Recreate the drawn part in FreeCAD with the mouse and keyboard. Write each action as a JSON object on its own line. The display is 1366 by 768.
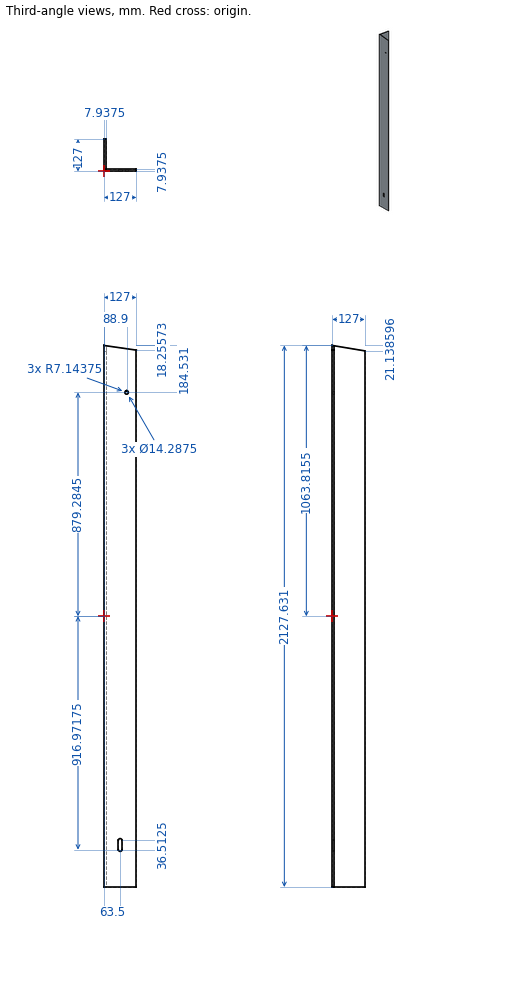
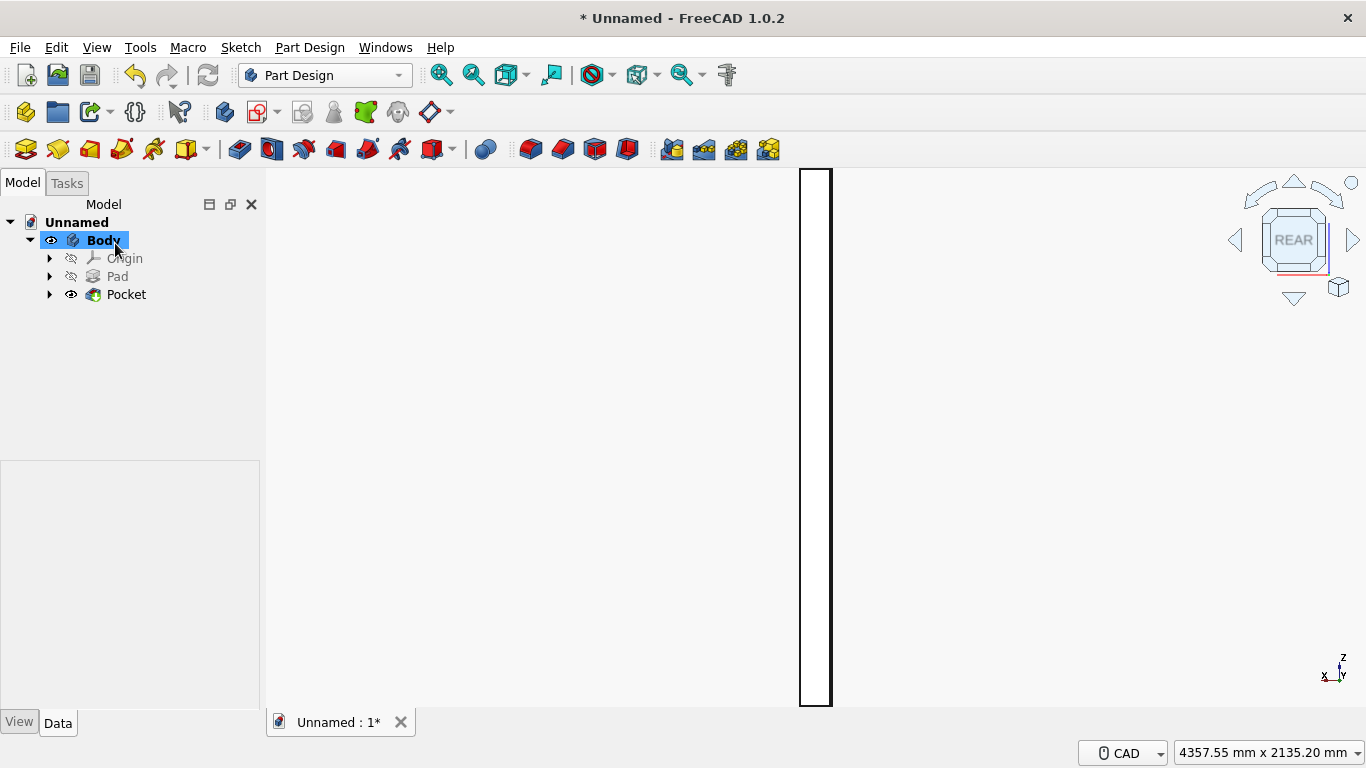
{"action": "left_click", "coordinate": [815, 207]}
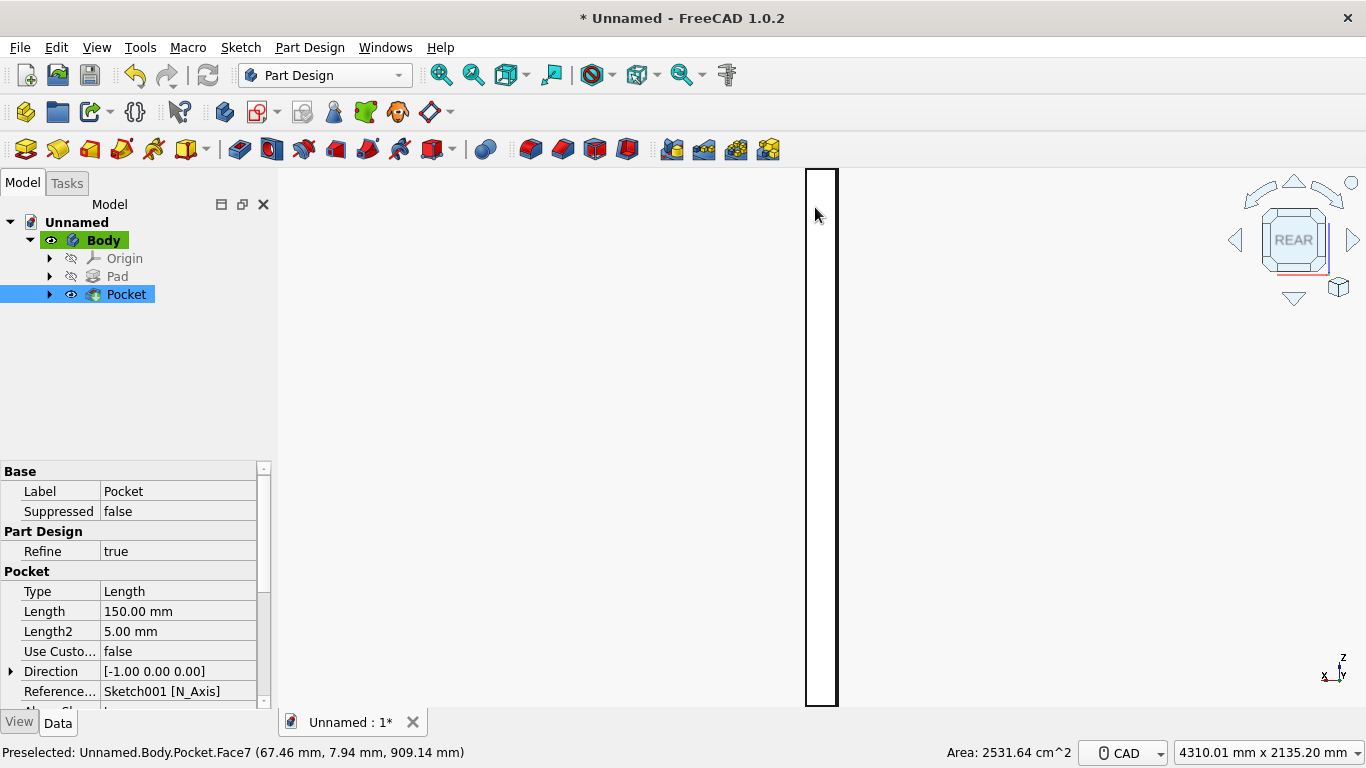
{"action": "left_click", "coordinate": [258, 112]}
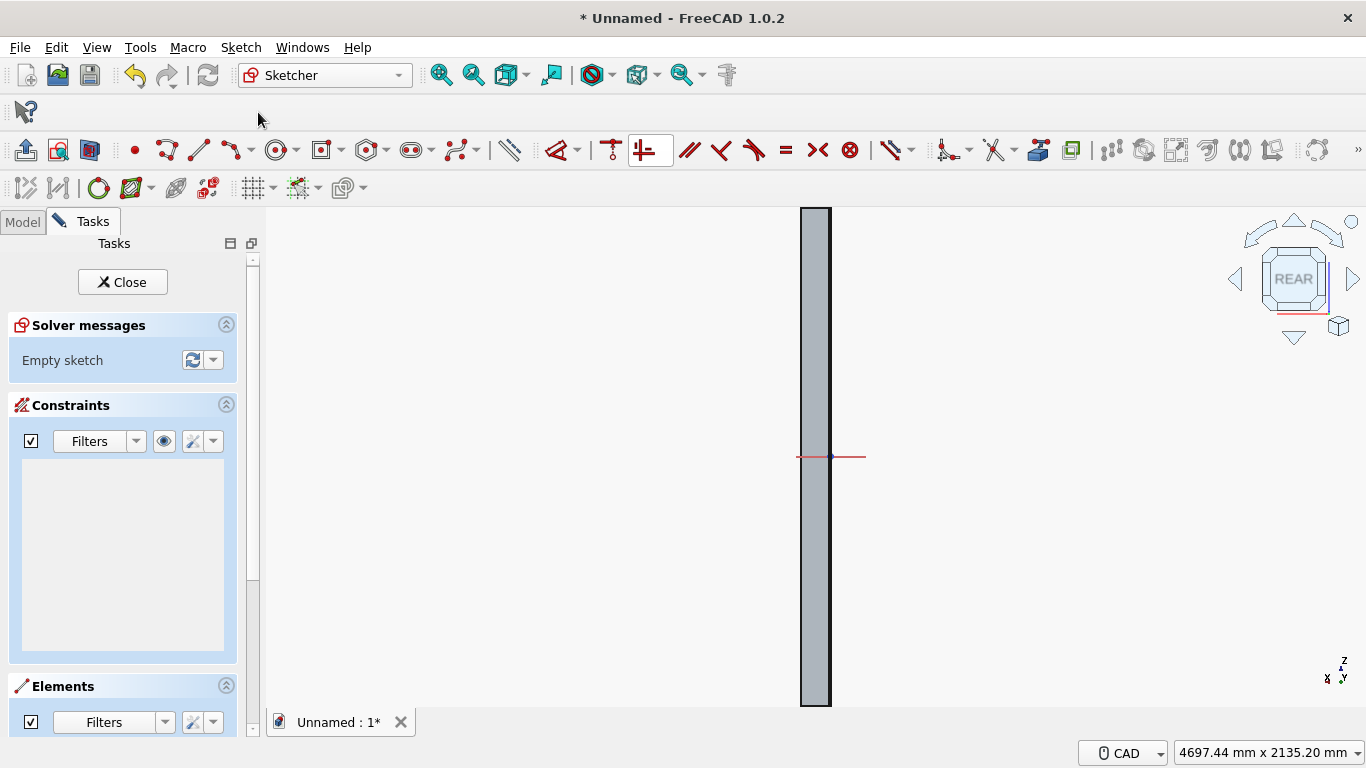
{"action": "scroll", "coordinate": [608, 490], "scroll_direction": "down", "scroll_amount": 2}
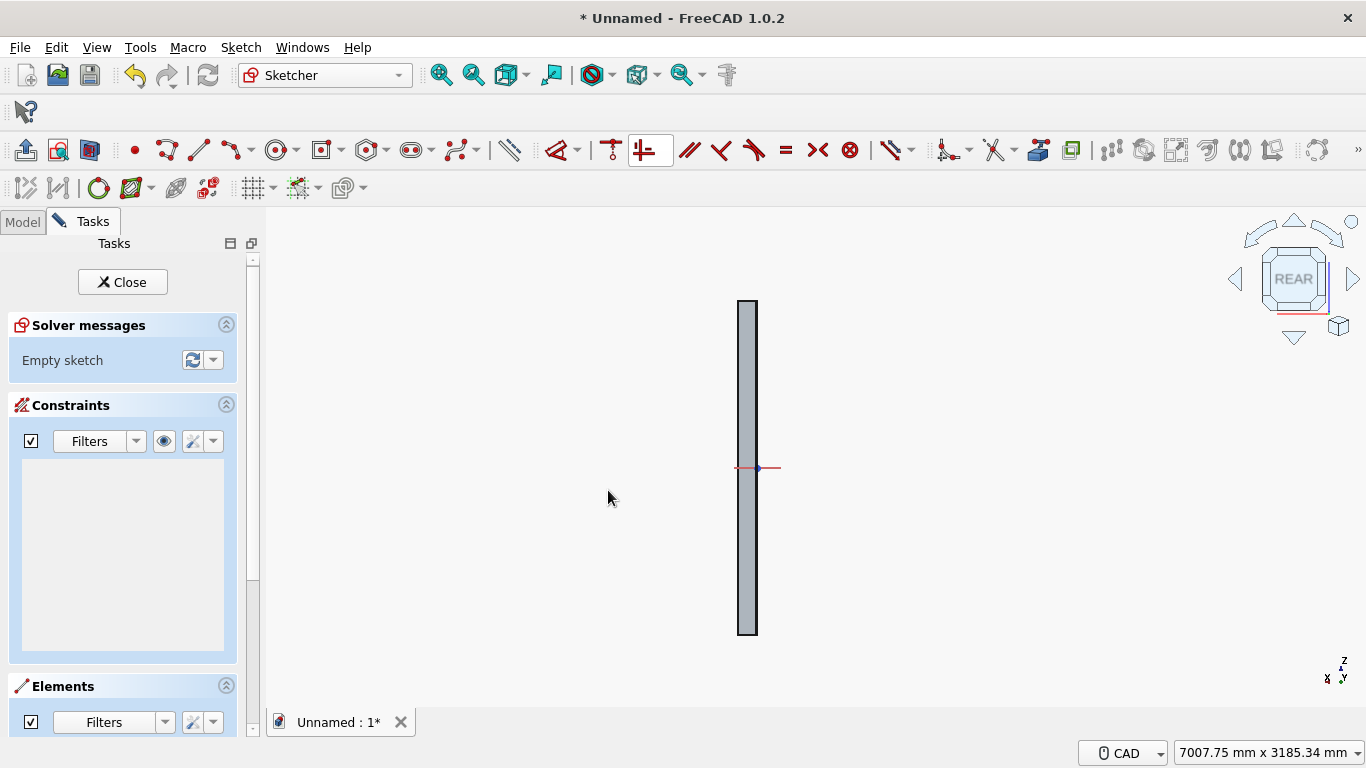
{"action": "left_click", "coordinate": [168, 150]}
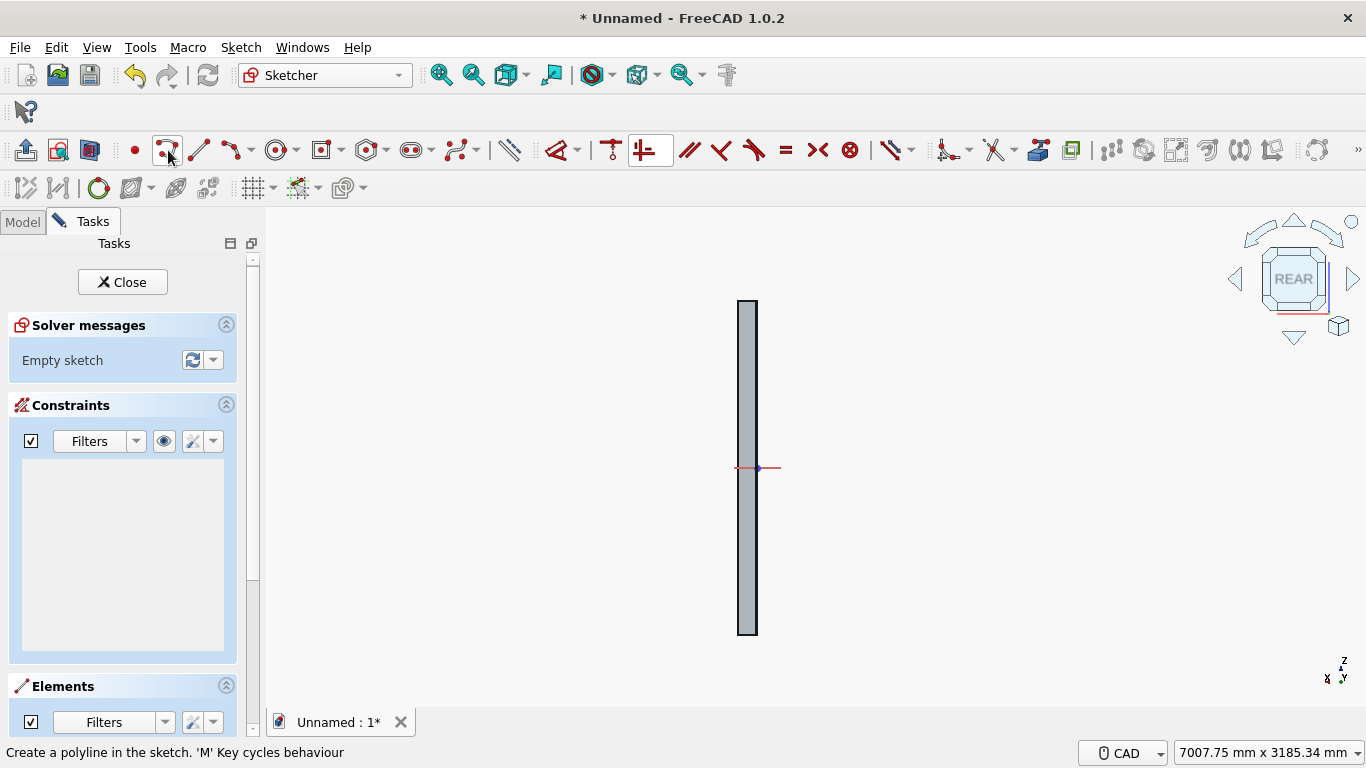
{"action": "left_click", "coordinate": [738, 304]}
{"action": "left_click", "coordinate": [757, 301]}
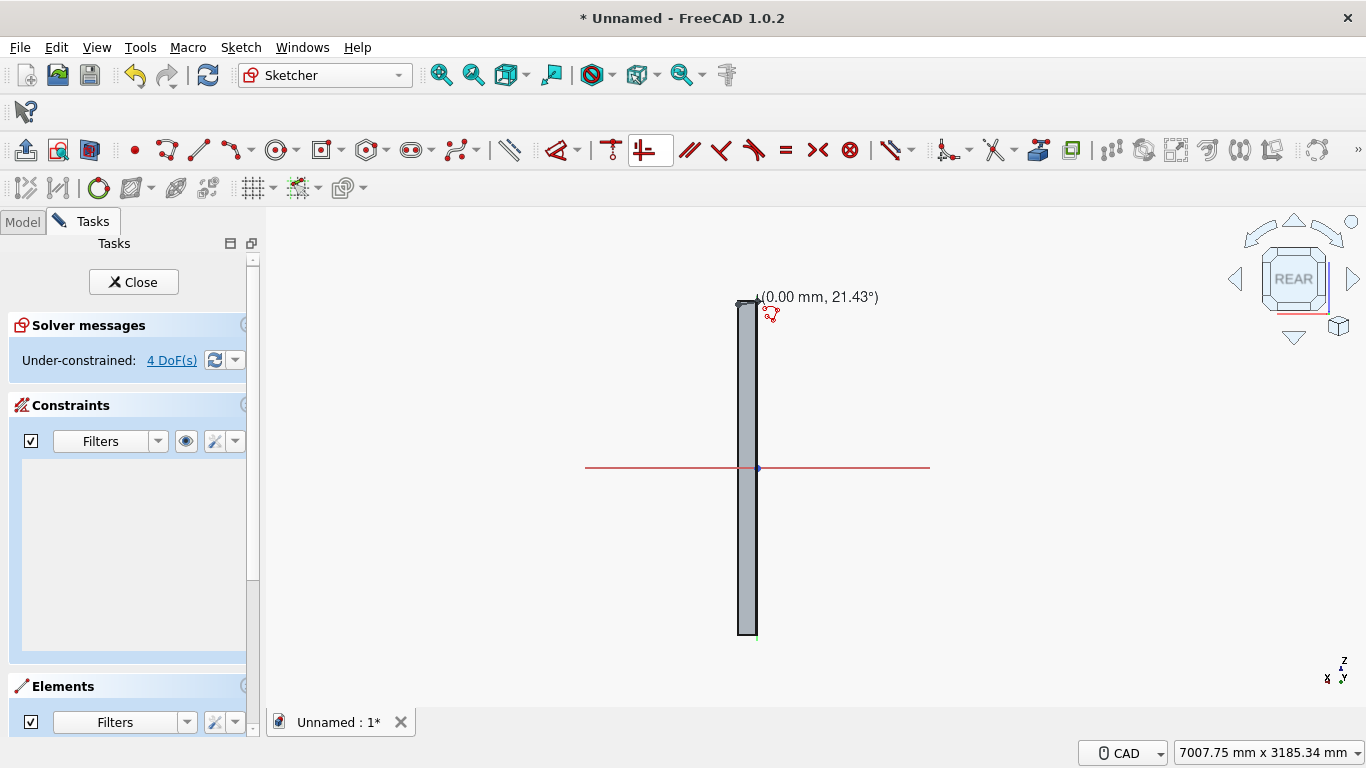
{"action": "scroll", "coordinate": [738, 301], "scroll_direction": "up", "scroll_amount": 9}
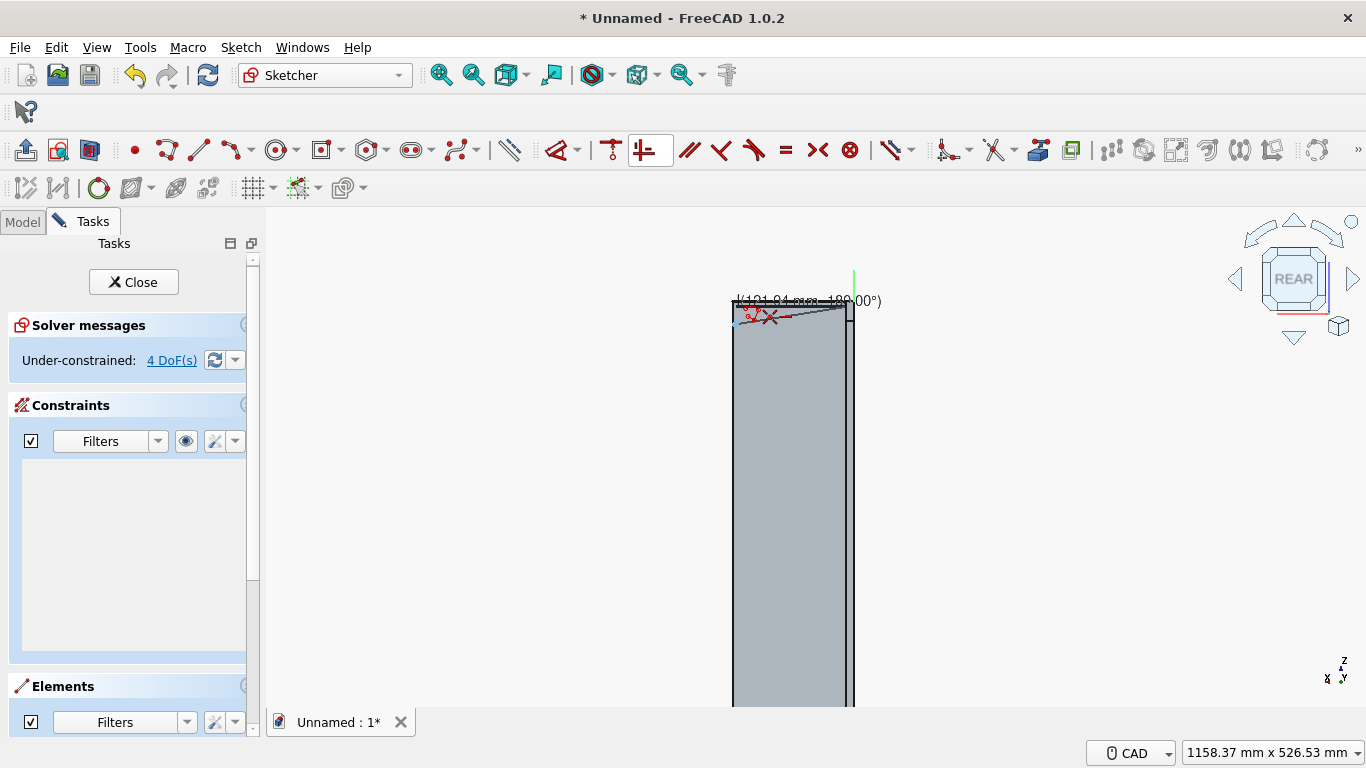
{"action": "left_click", "coordinate": [733, 300]}
{"action": "left_click", "coordinate": [736, 324]}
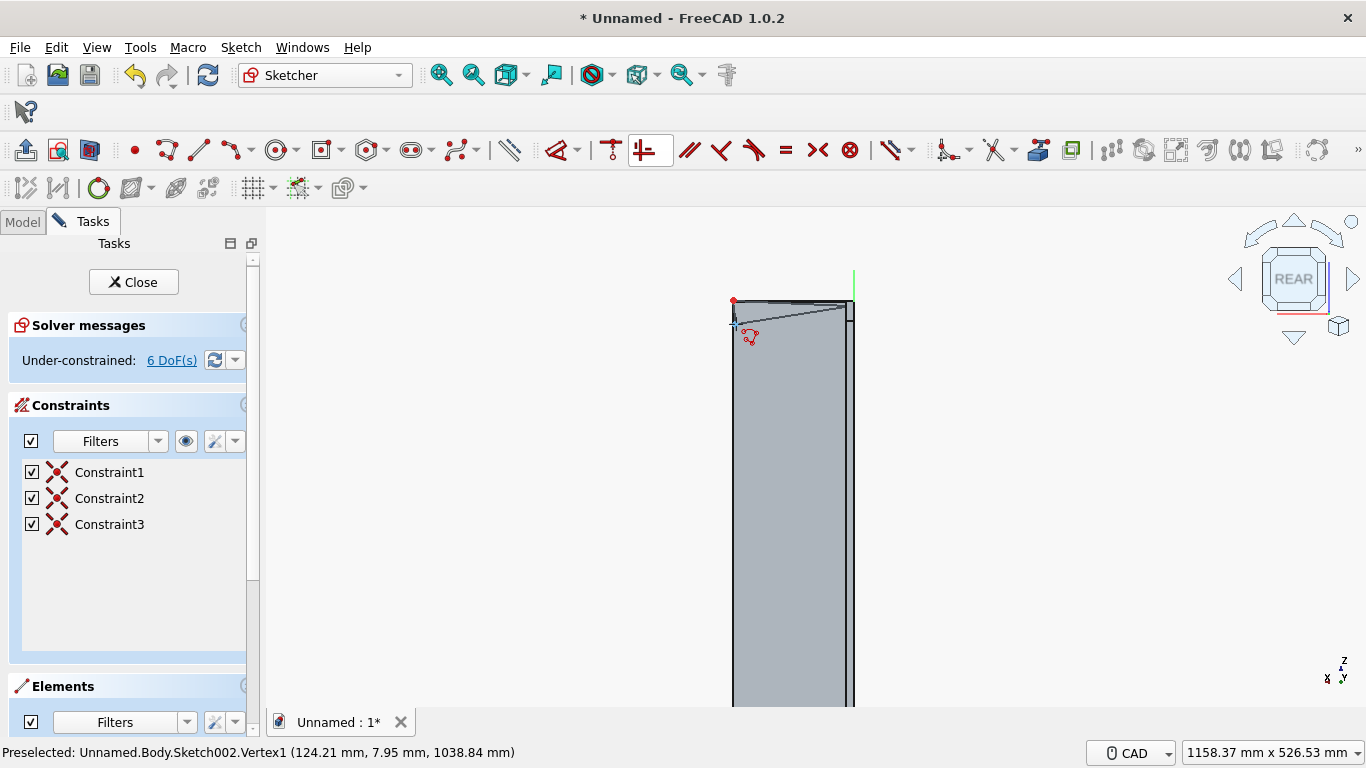
{"action": "left_click", "coordinate": [412, 150]}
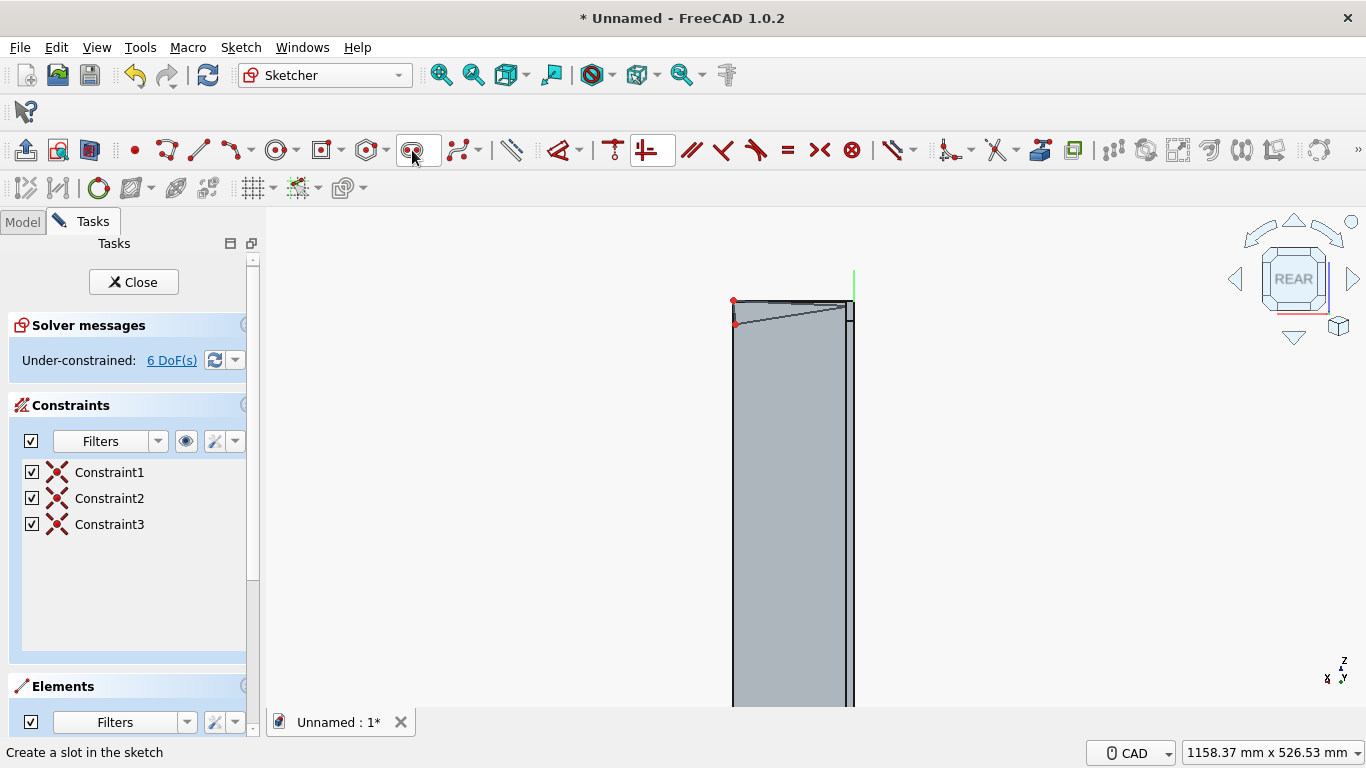
{"action": "scroll", "coordinate": [738, 301], "scroll_direction": "down", "scroll_amount": 9}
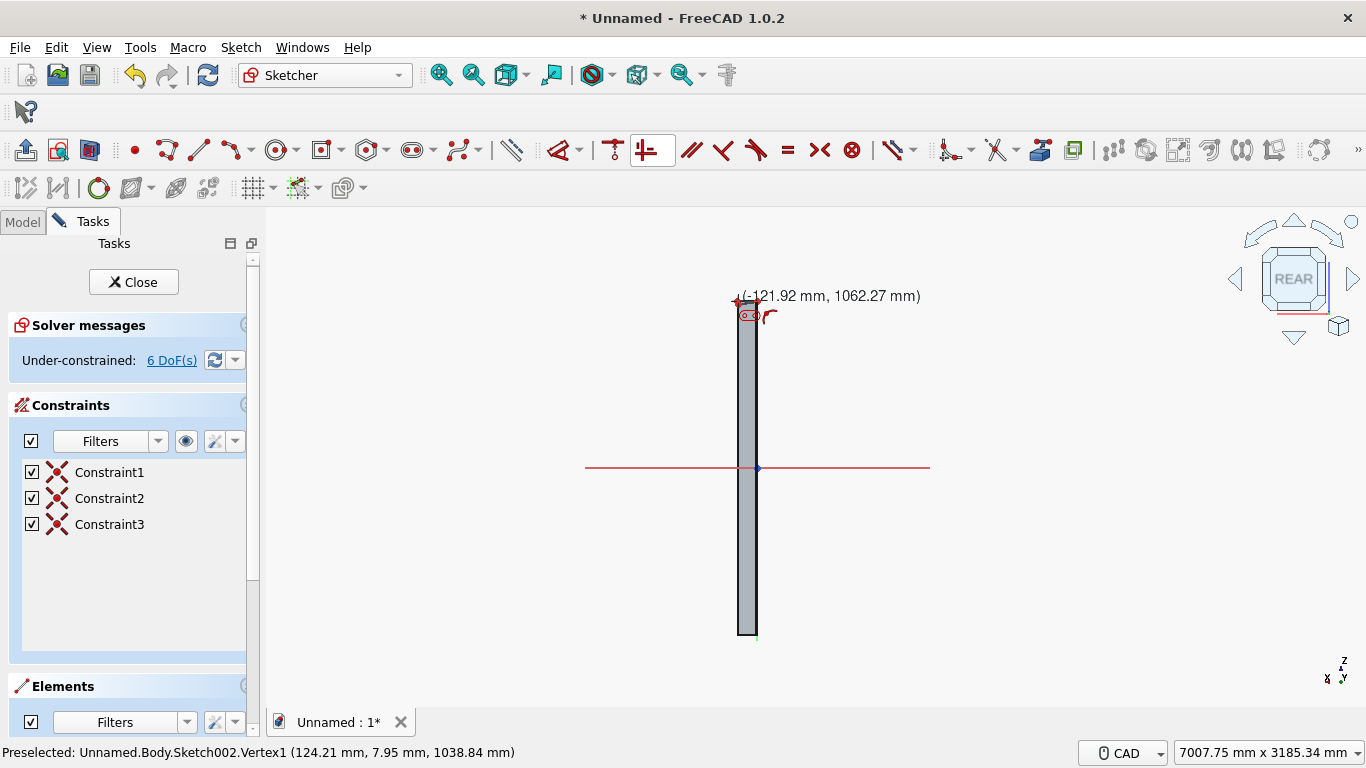
{"action": "scroll", "coordinate": [748, 612], "scroll_direction": "up", "scroll_amount": 16}